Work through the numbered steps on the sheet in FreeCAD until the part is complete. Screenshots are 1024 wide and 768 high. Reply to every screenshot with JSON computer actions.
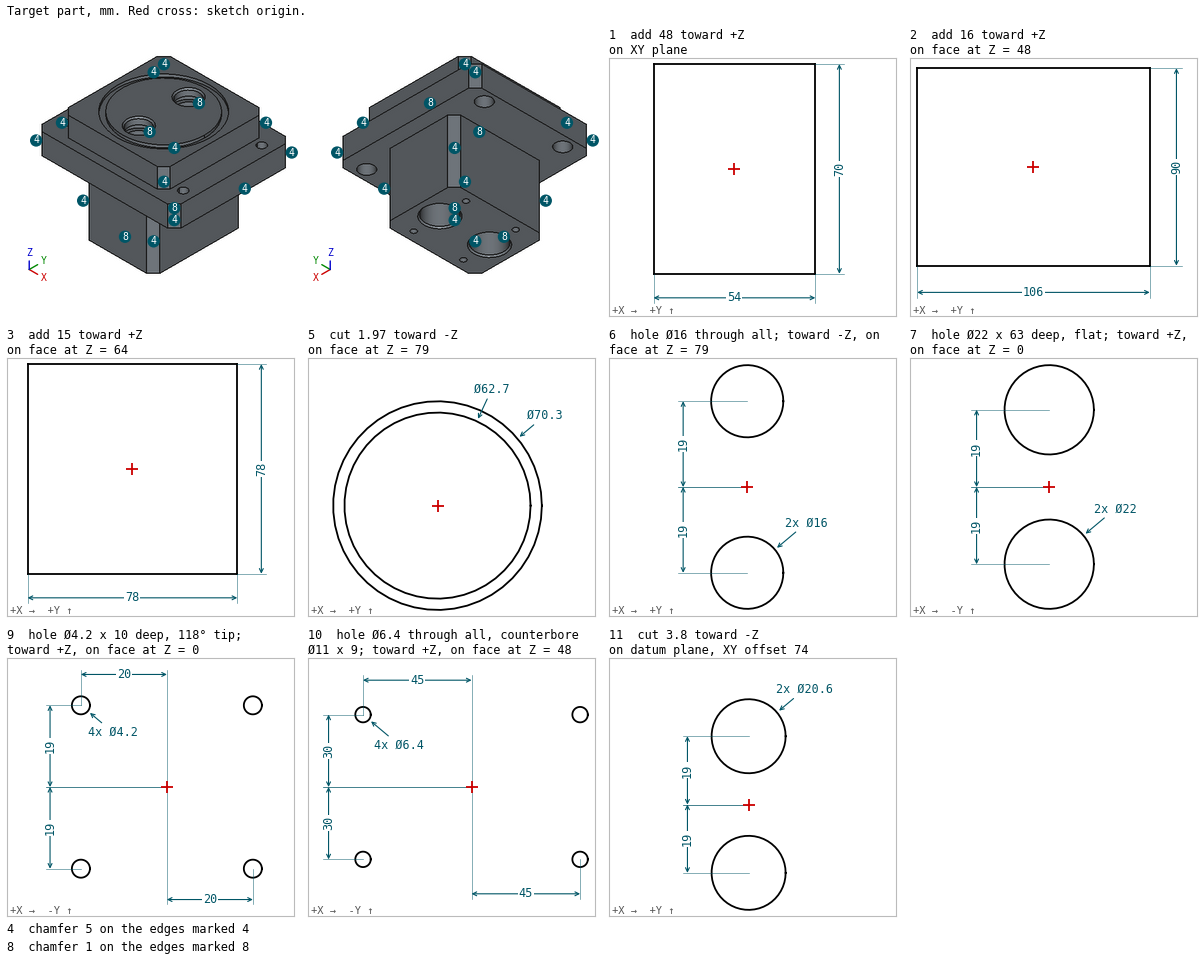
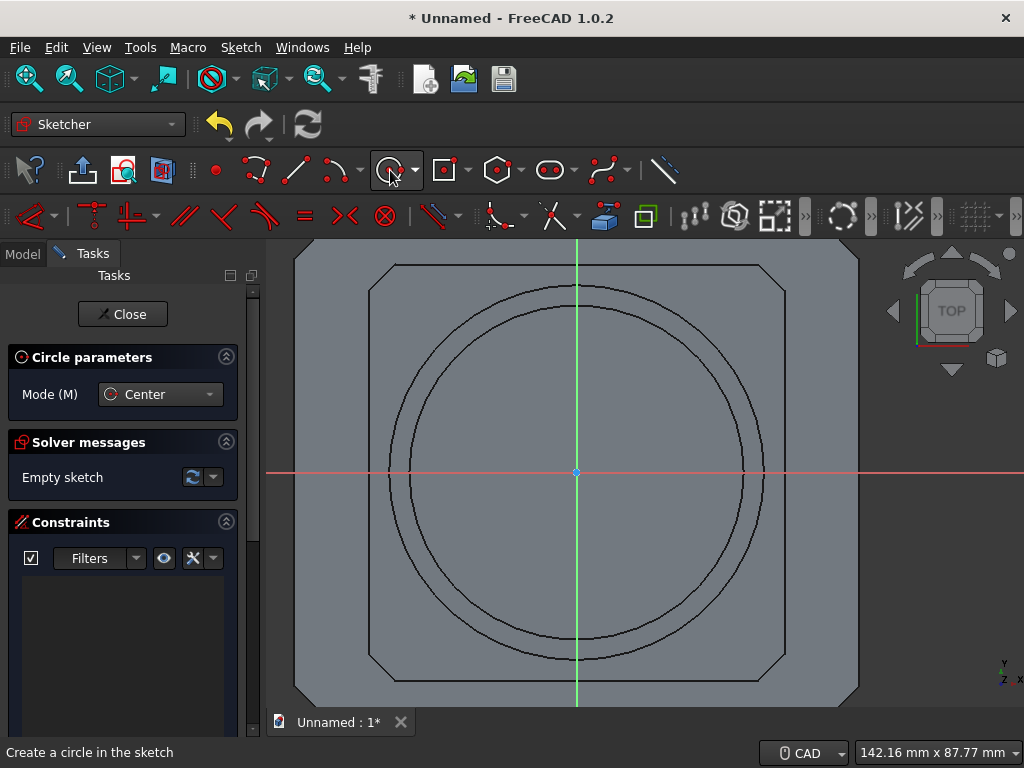
{"action": "left_click", "coordinate": [577, 574]}
{"action": "mouse_move", "coordinate": [607, 544]}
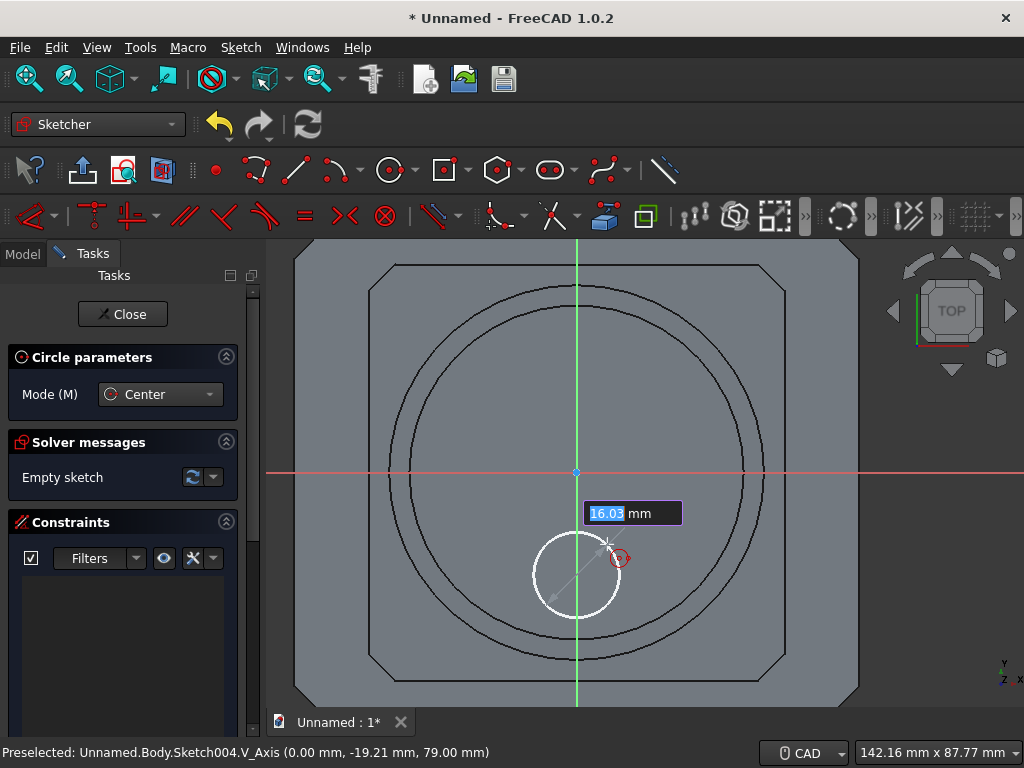
{"action": "type", "text": "16"}
{"action": "key", "text": "Return"}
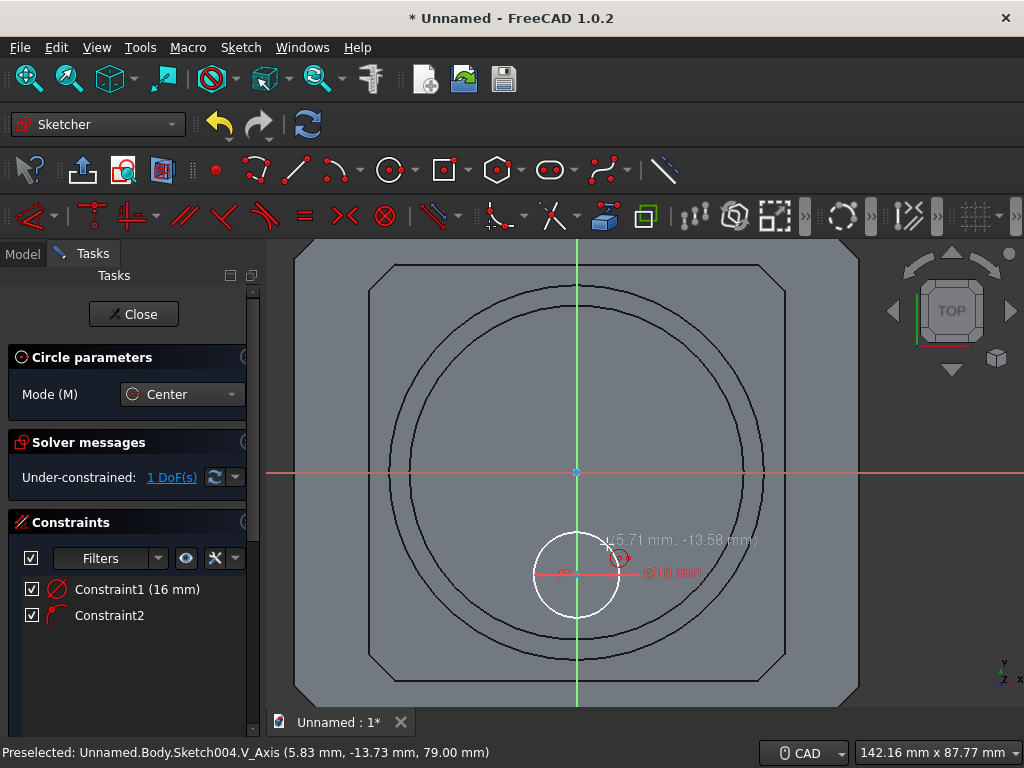
{"action": "left_click", "coordinate": [577, 371]}
{"action": "mouse_move", "coordinate": [607, 341]}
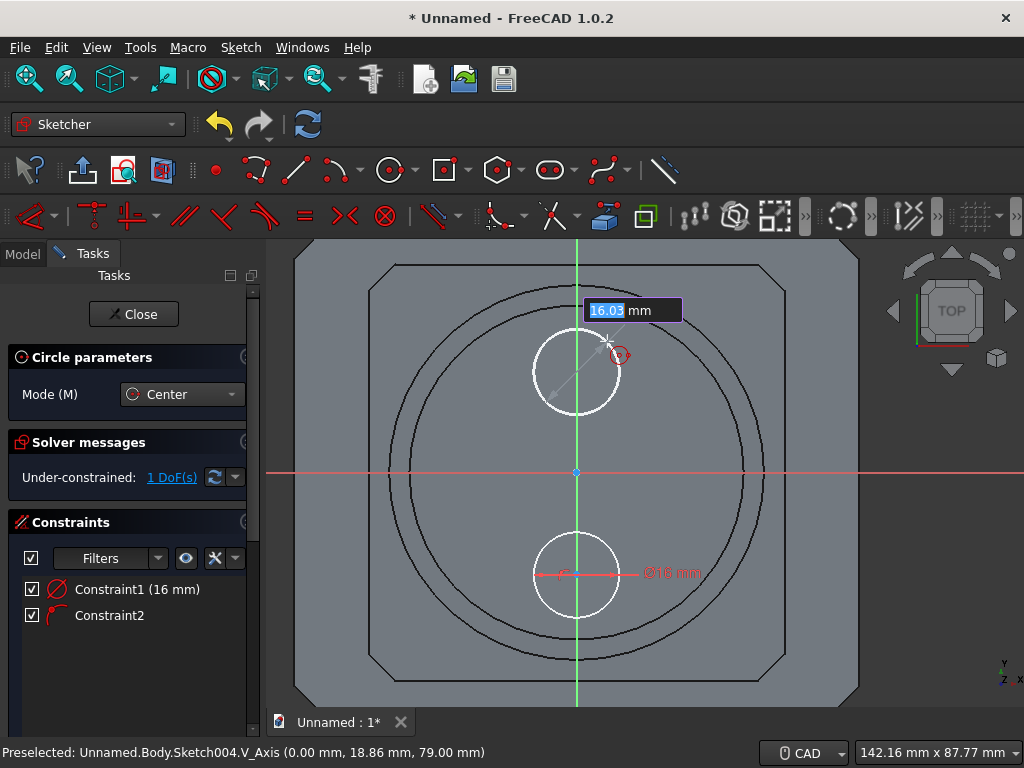
{"action": "type", "text": "16"}
{"action": "key", "text": "Return"}
{"action": "key", "text": "Escape"}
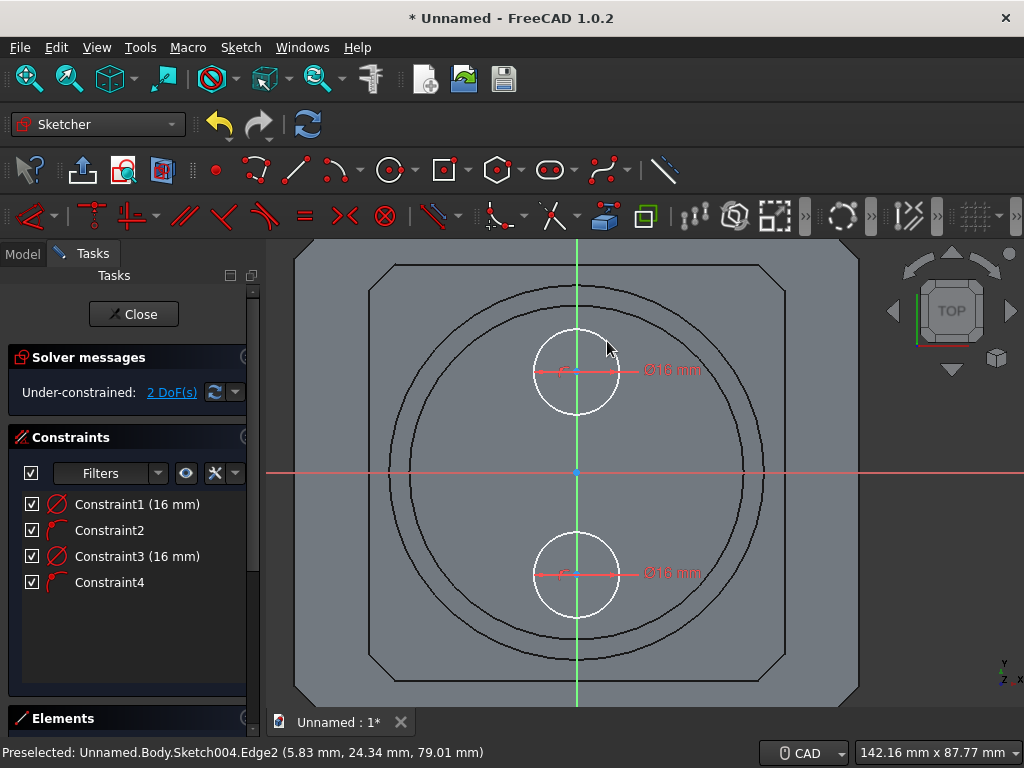
{"action": "left_click", "coordinate": [30, 216]}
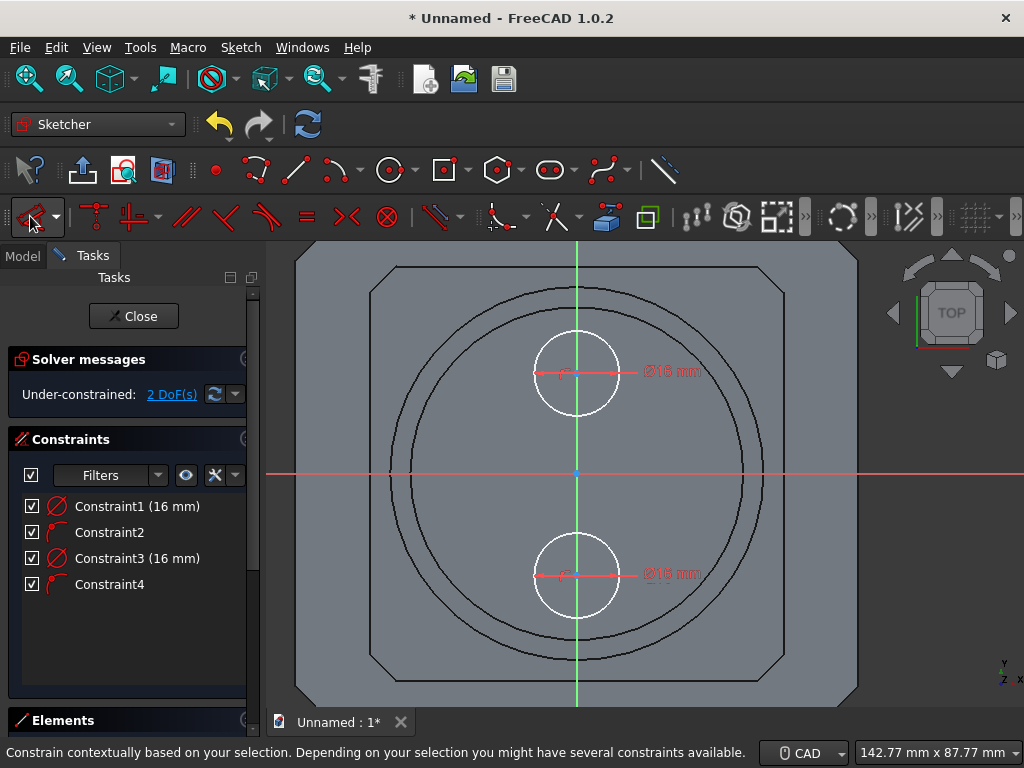
{"action": "left_click", "coordinate": [577, 576]}
{"action": "left_click", "coordinate": [611, 525]}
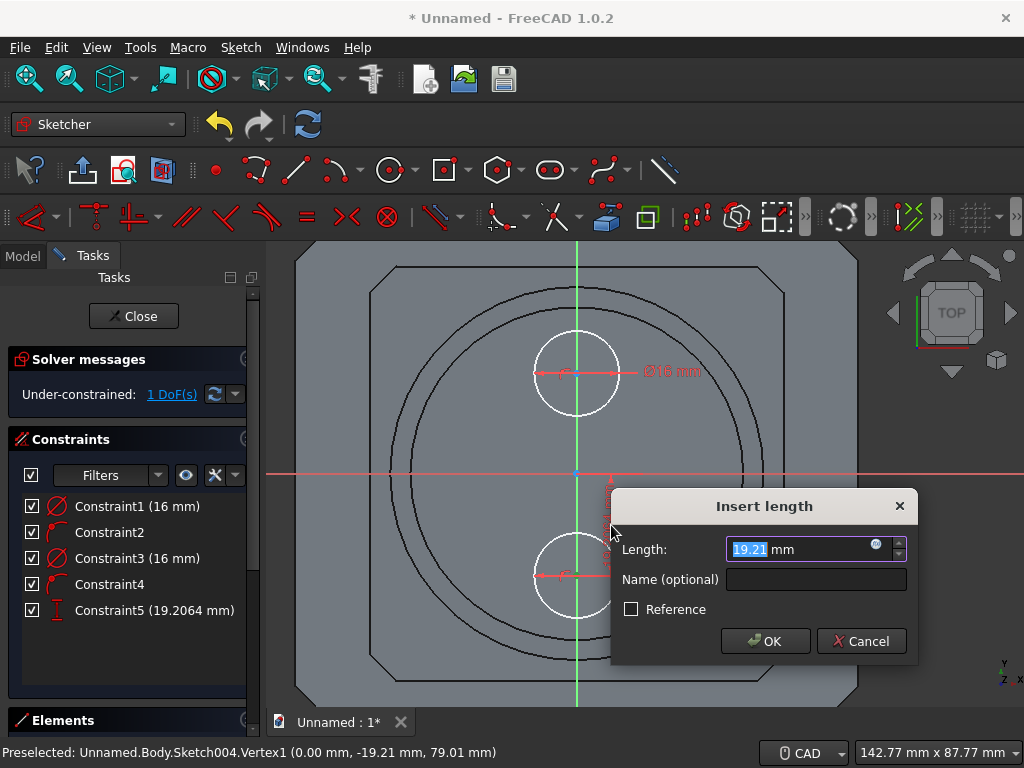
{"action": "type", "text": "19"}
{"action": "key", "text": "Return"}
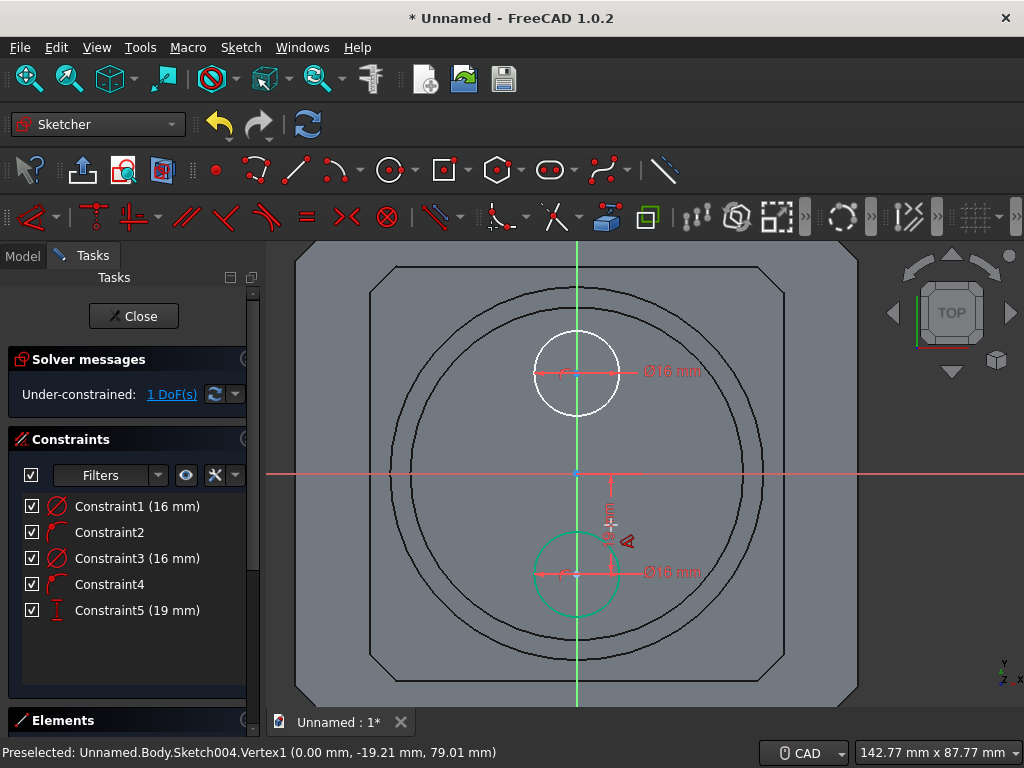
{"action": "left_click", "coordinate": [577, 373]}
{"action": "left_click", "coordinate": [611, 424]}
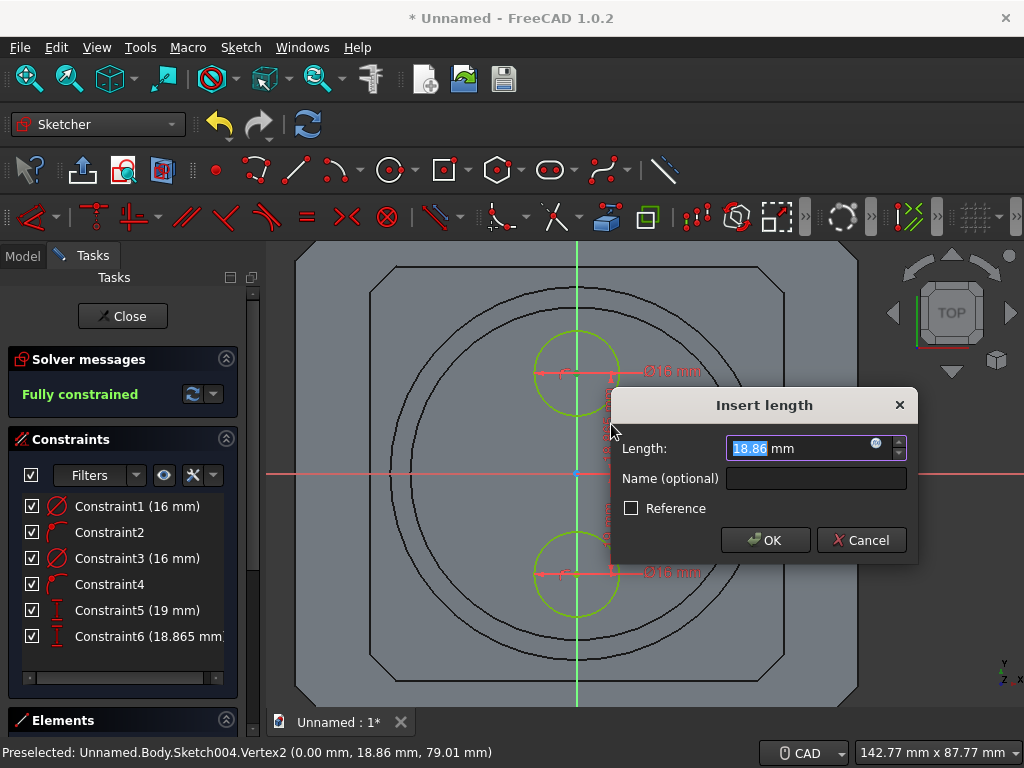
{"action": "type", "text": "19"}
{"action": "key", "text": "Return"}
{"action": "key", "text": "Escape"}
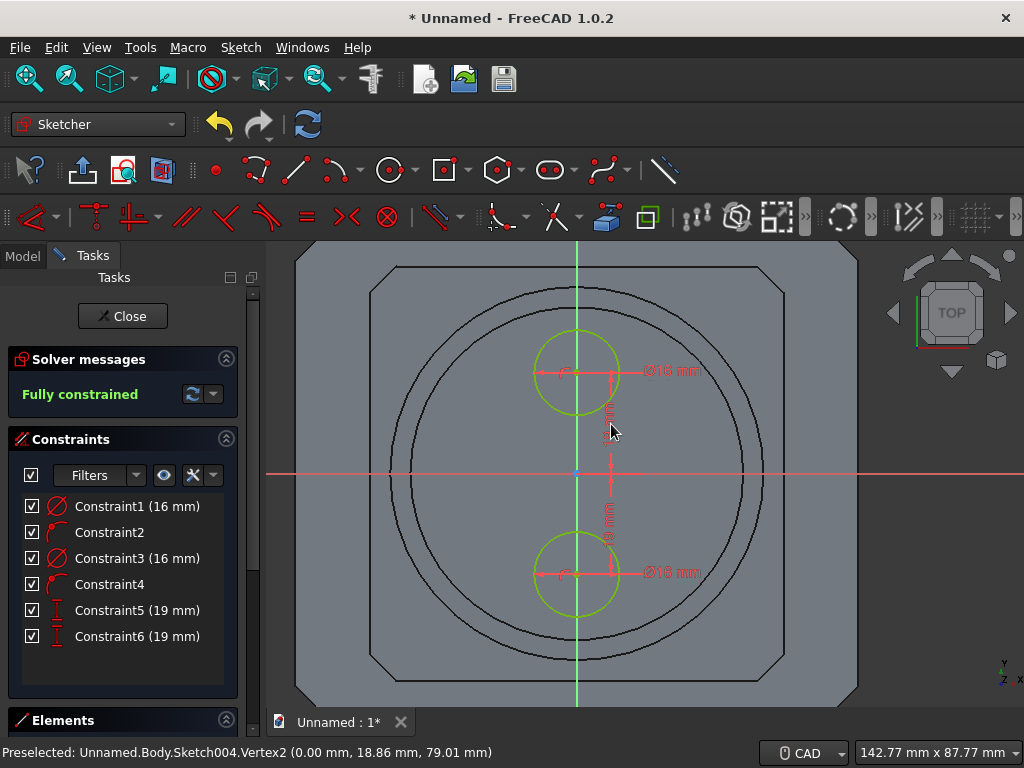
{"action": "left_click", "coordinate": [123, 316]}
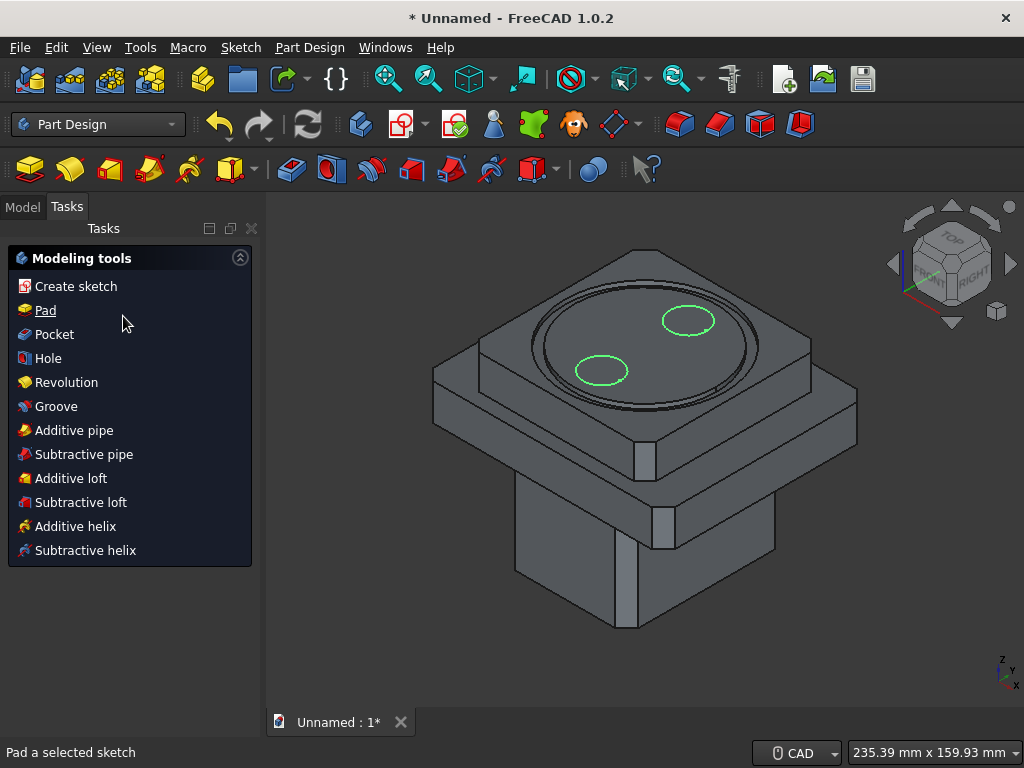
{"action": "left_click", "coordinate": [332, 170]}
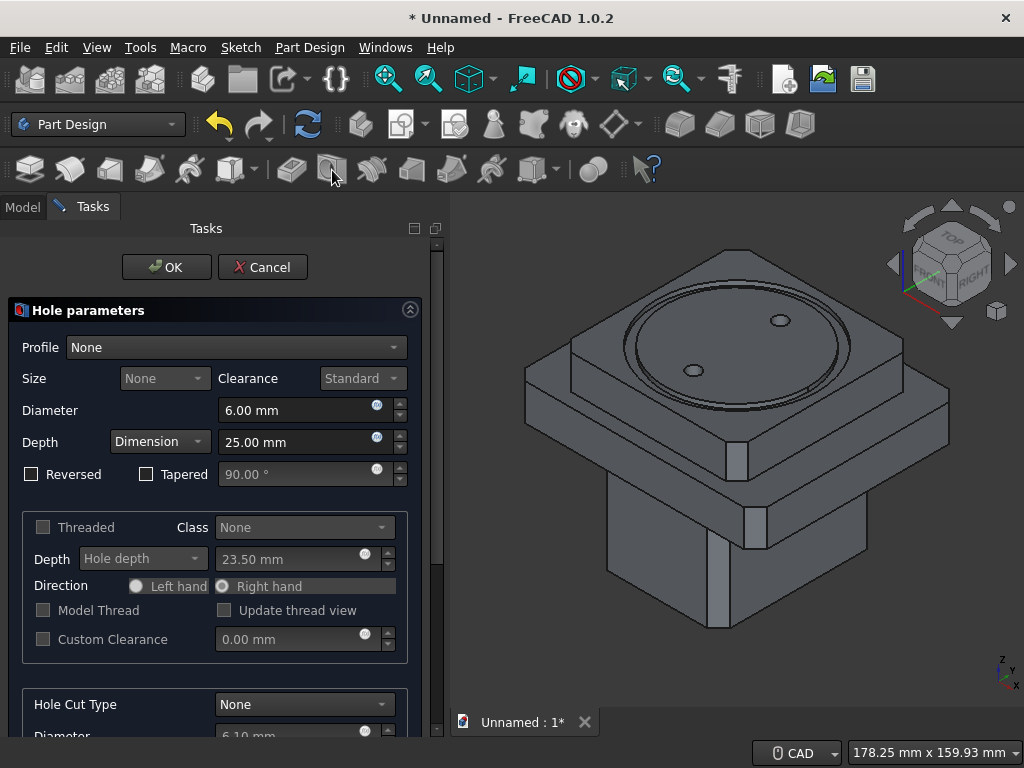
{"action": "triple_click", "coordinate": [305, 410]}